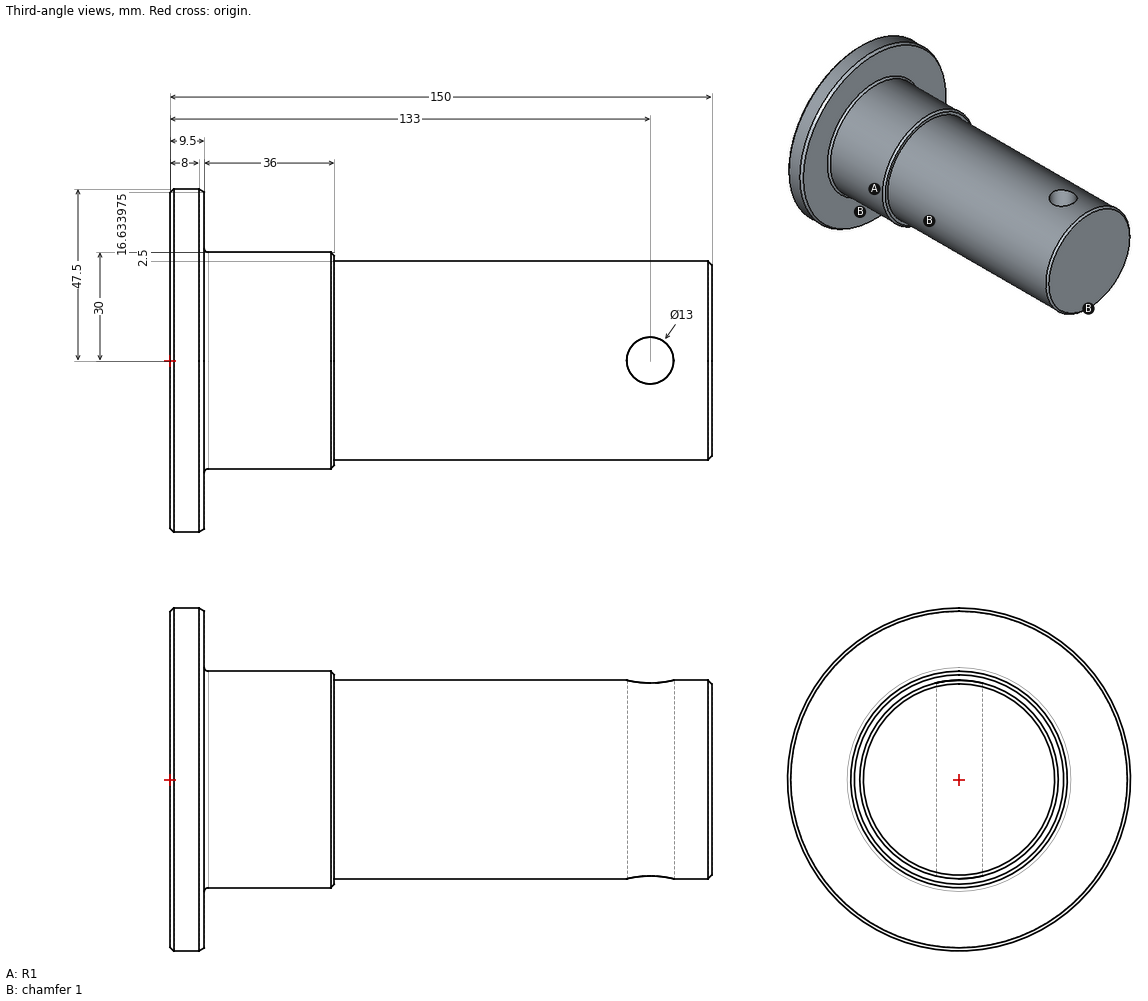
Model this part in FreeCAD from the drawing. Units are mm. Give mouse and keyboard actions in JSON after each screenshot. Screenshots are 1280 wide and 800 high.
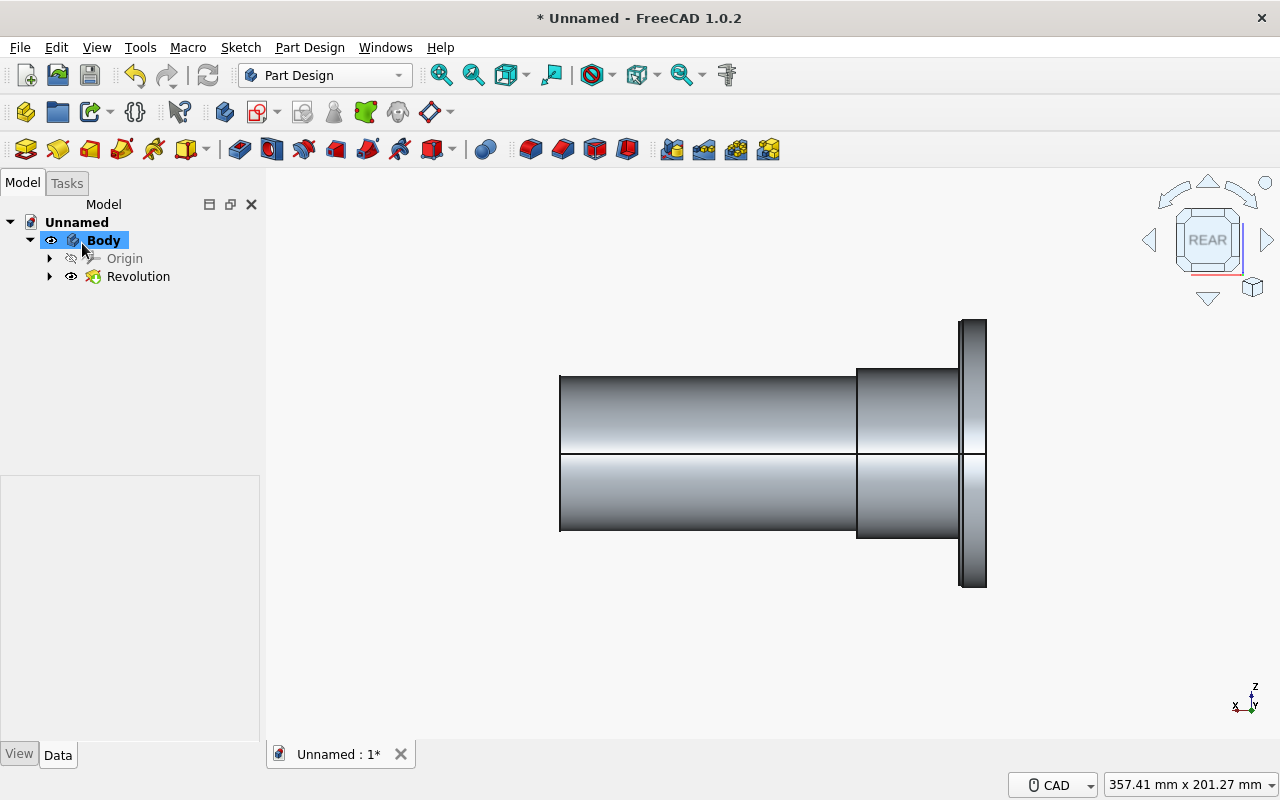
{"action": "key", "text": "6"}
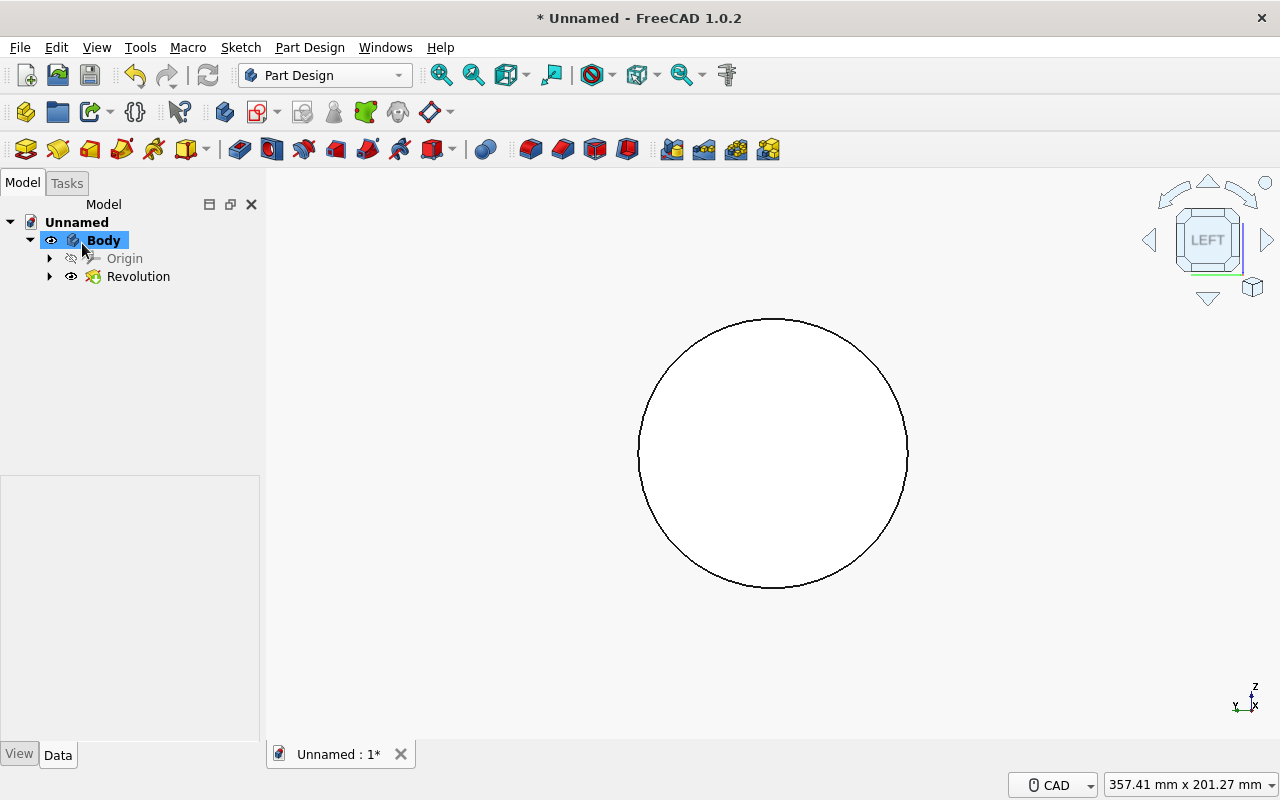
{"action": "key", "text": "v 3"}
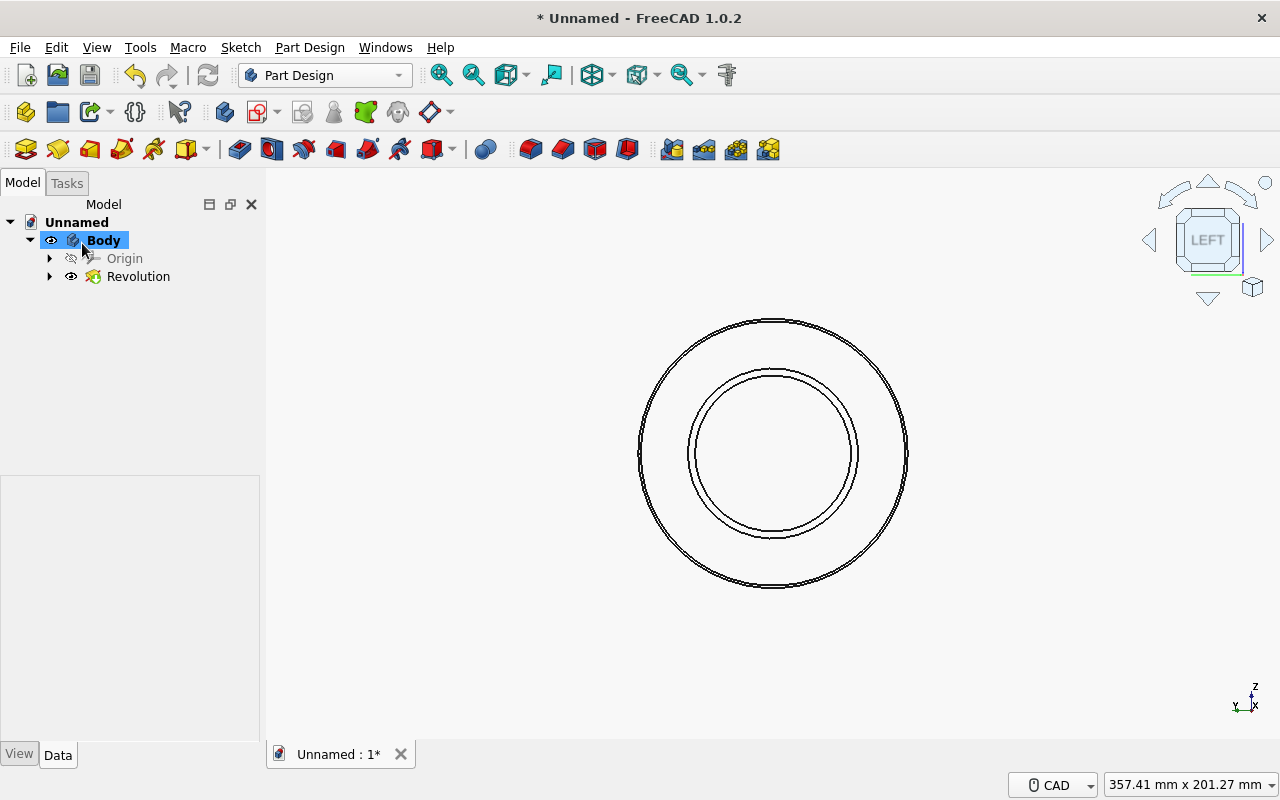
{"action": "key", "text": "0"}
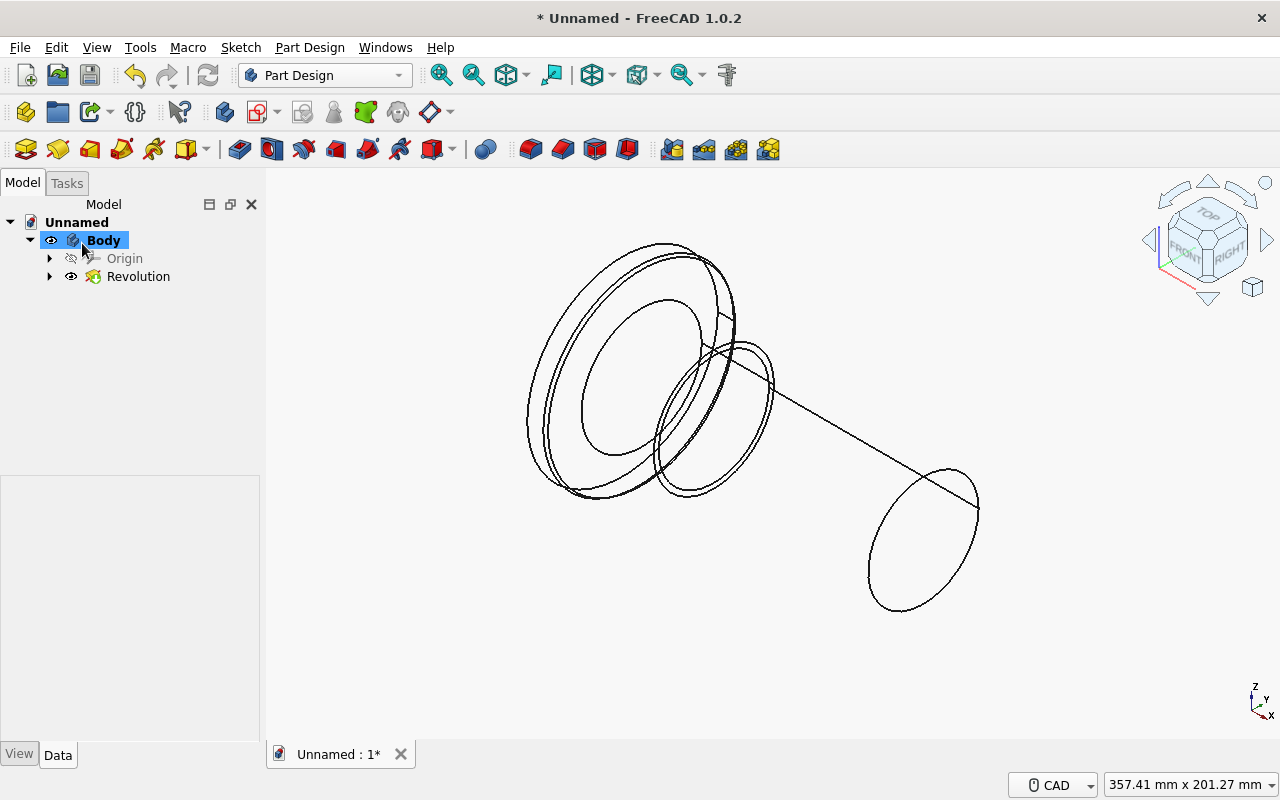
{"action": "left_click", "coordinate": [581, 411]}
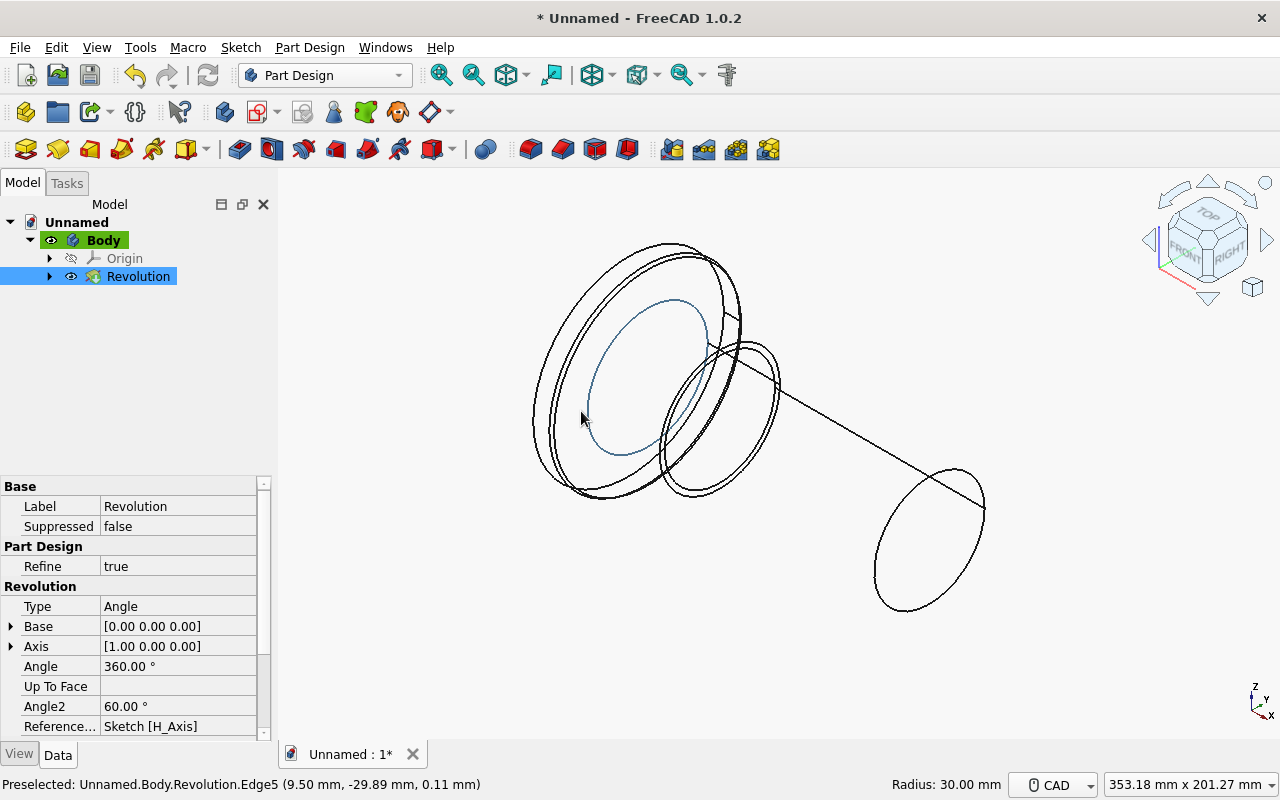
{"action": "key", "text": "v 1"}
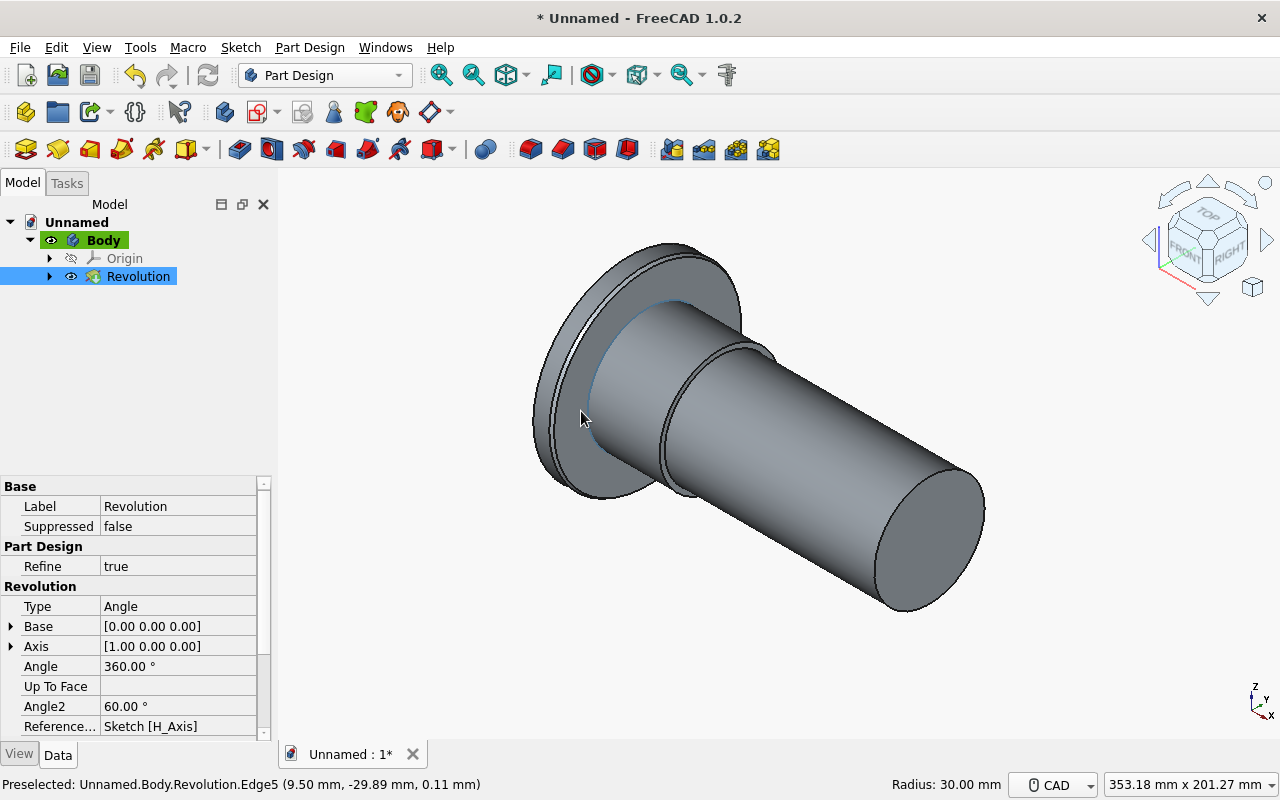
{"action": "left_click", "coordinate": [532, 150]}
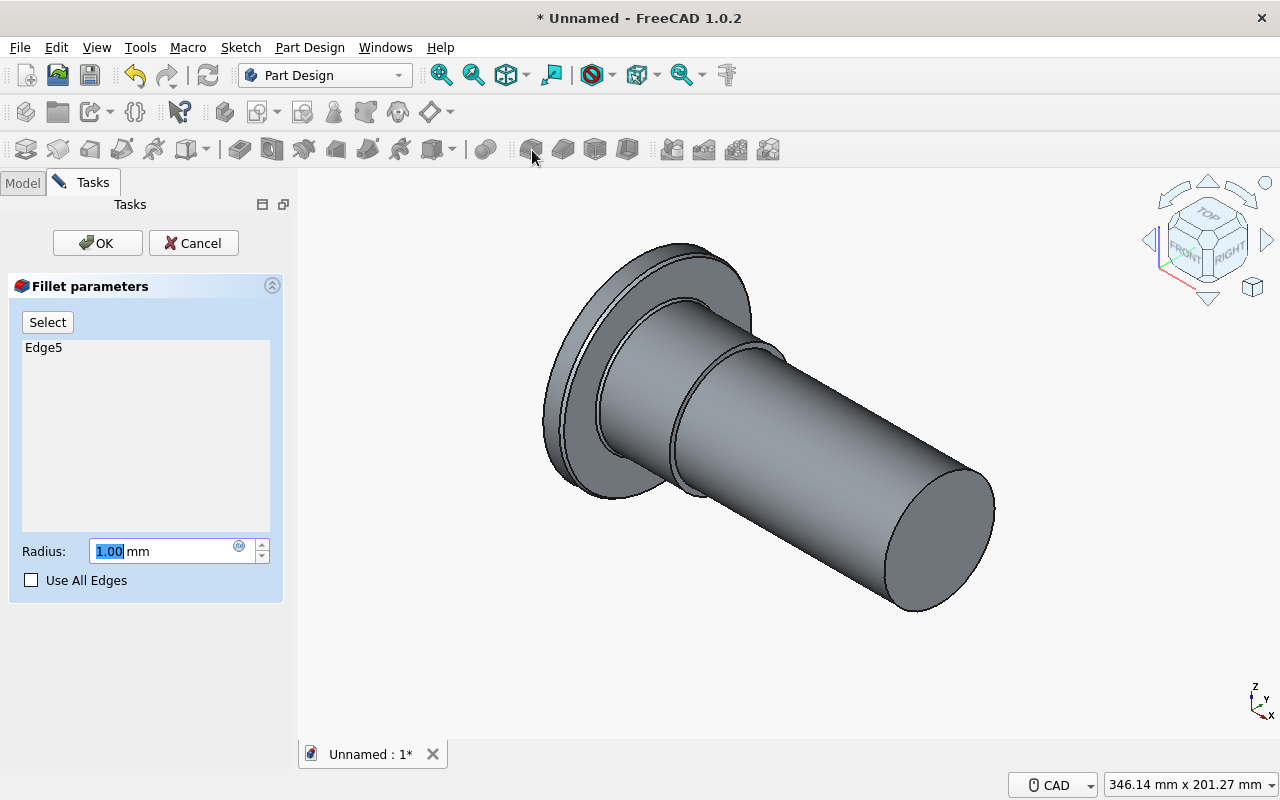
{"action": "type", "text": "1"}
{"action": "key", "text": "Tab"}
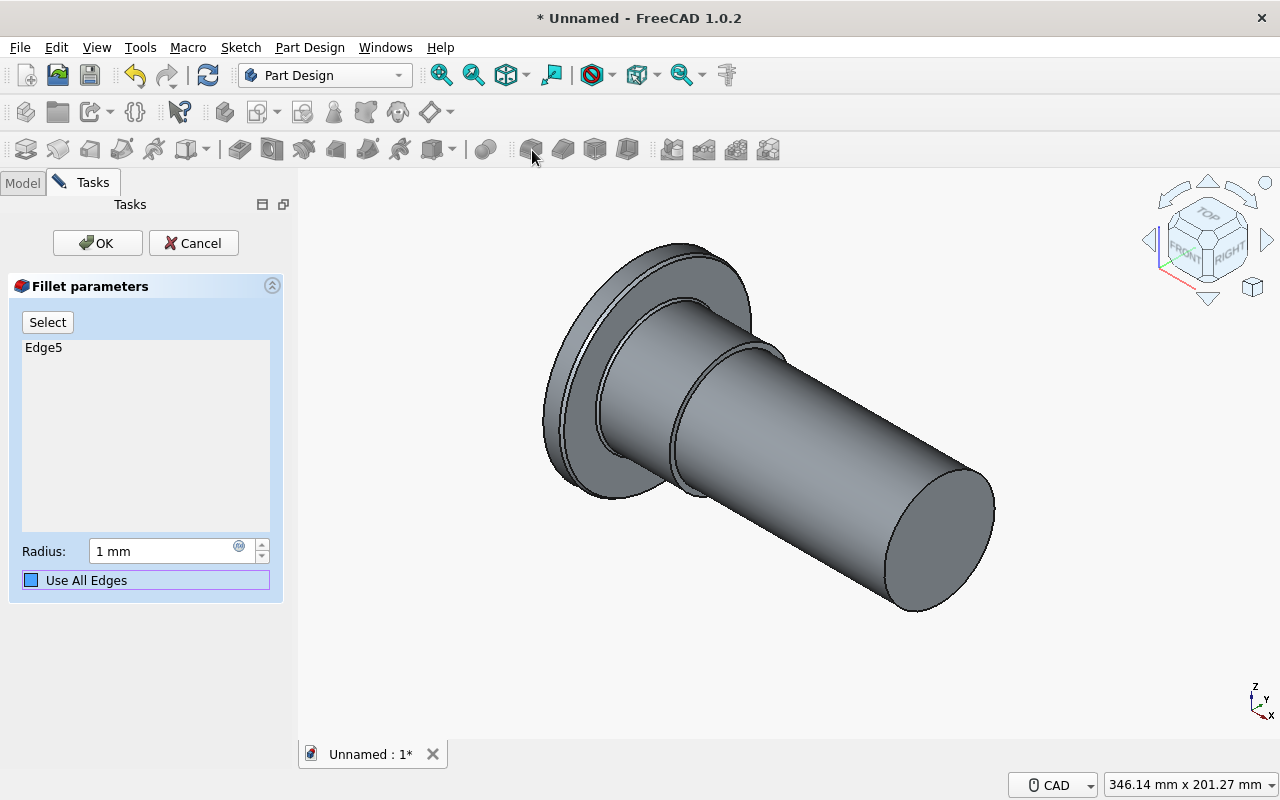
{"action": "left_click", "coordinate": [98, 243]}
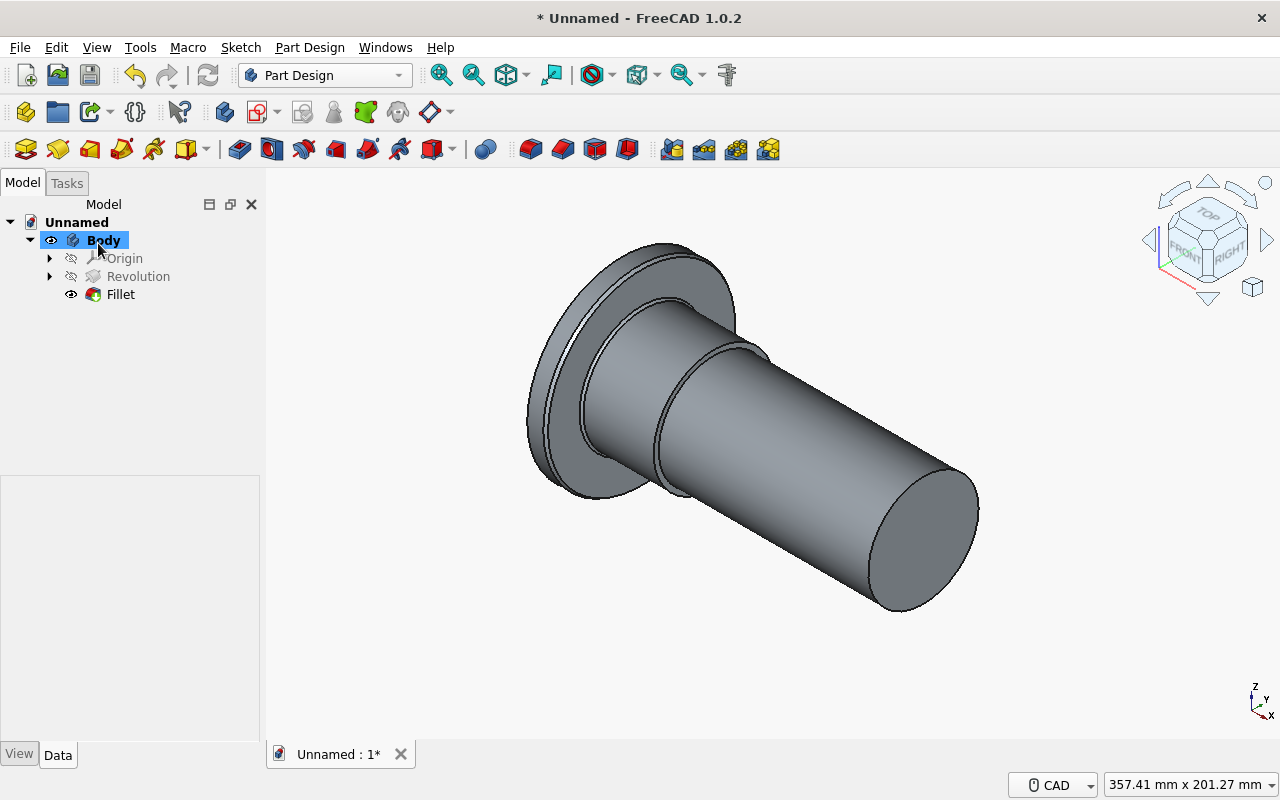
{"action": "left_click", "coordinate": [868, 571]}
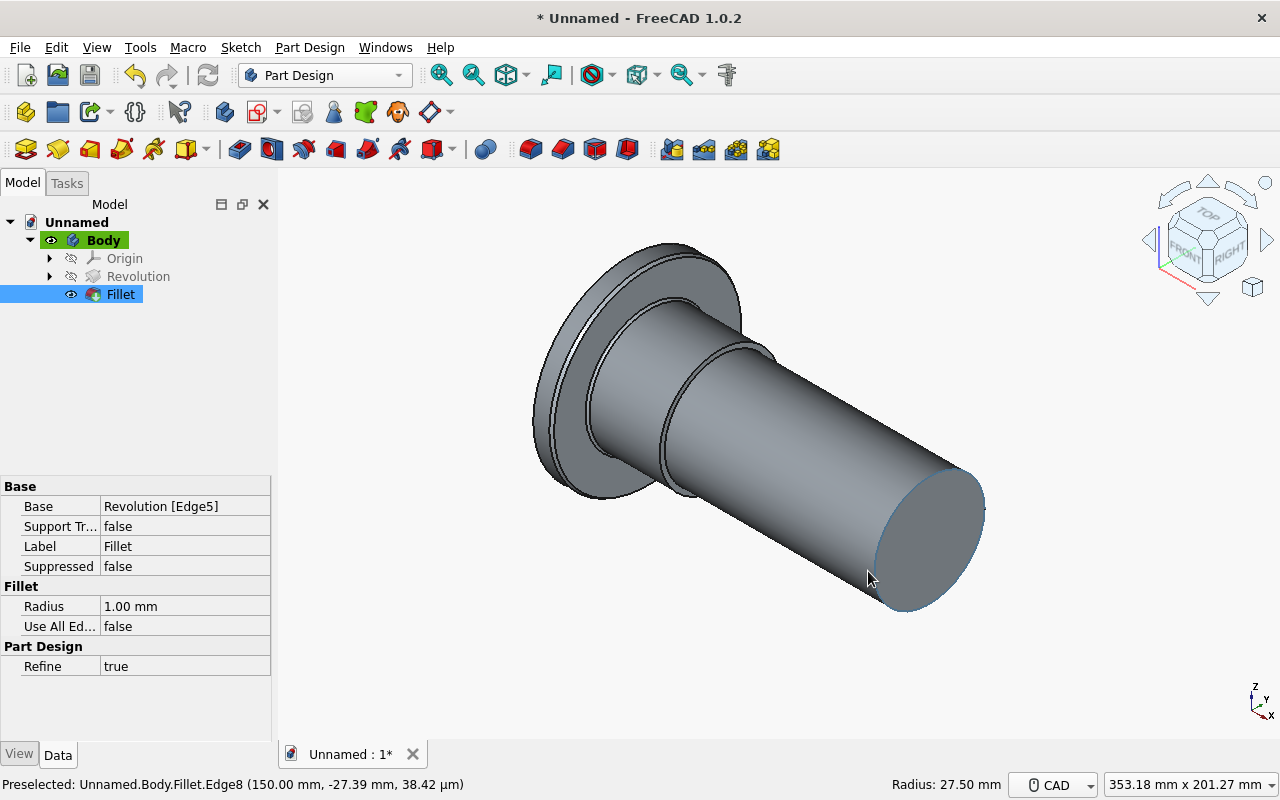
{"action": "left_click", "coordinate": [660, 453], "text": "ctrl"}